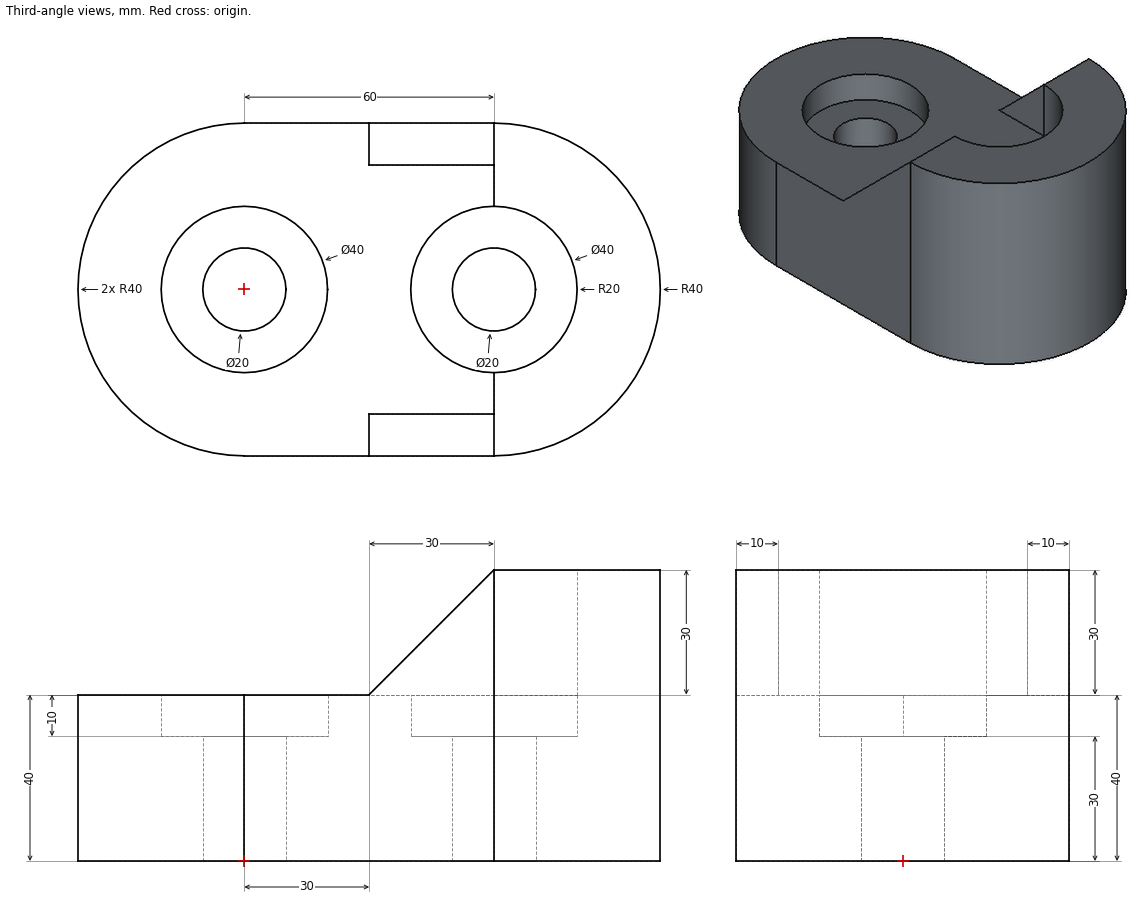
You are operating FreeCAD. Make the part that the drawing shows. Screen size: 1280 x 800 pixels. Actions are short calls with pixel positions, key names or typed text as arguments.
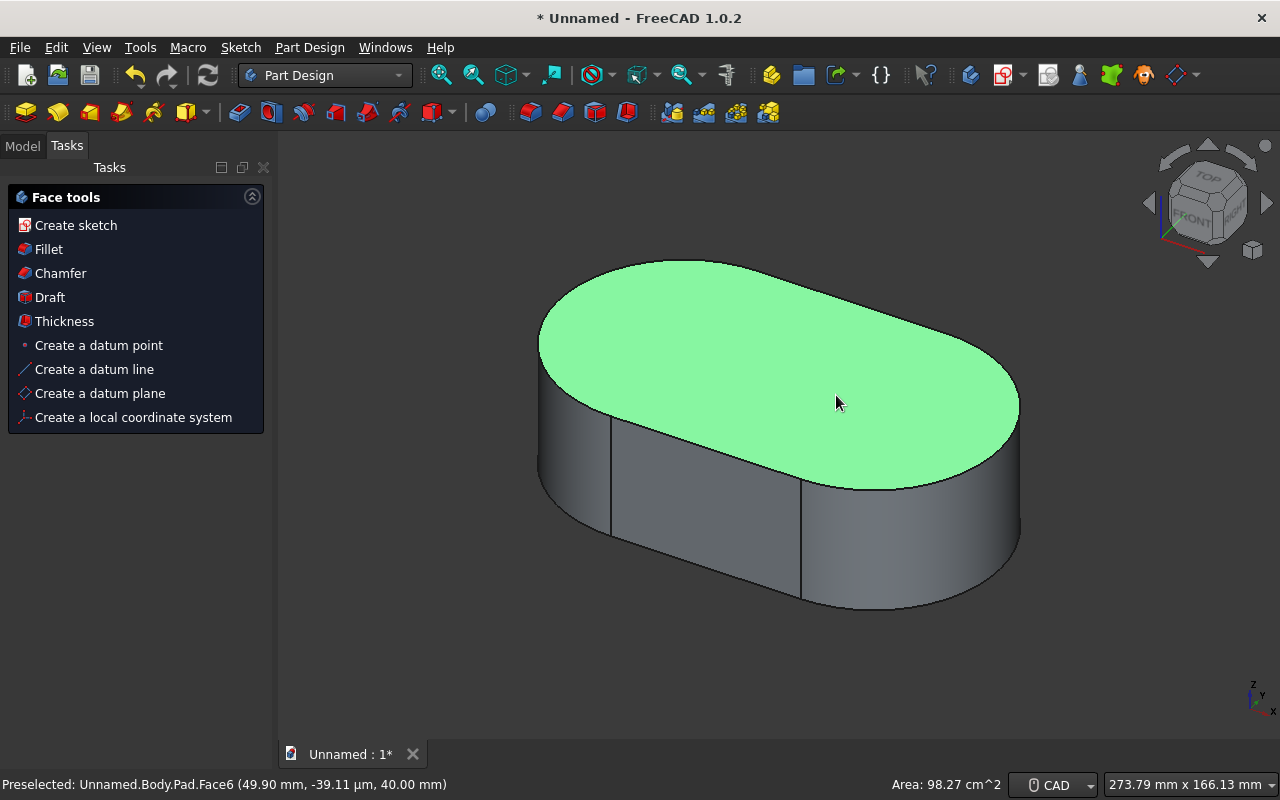
click(1004, 76)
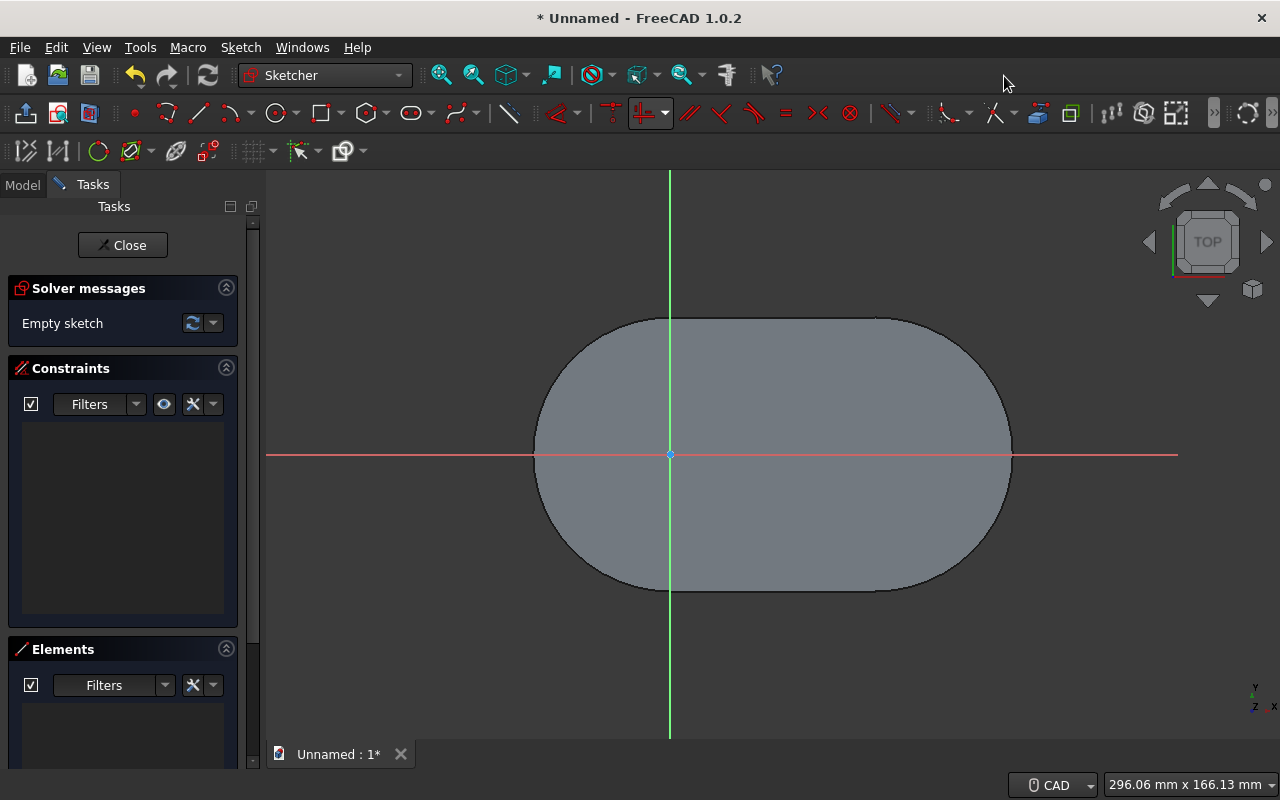
scroll(650, 454, up, 5)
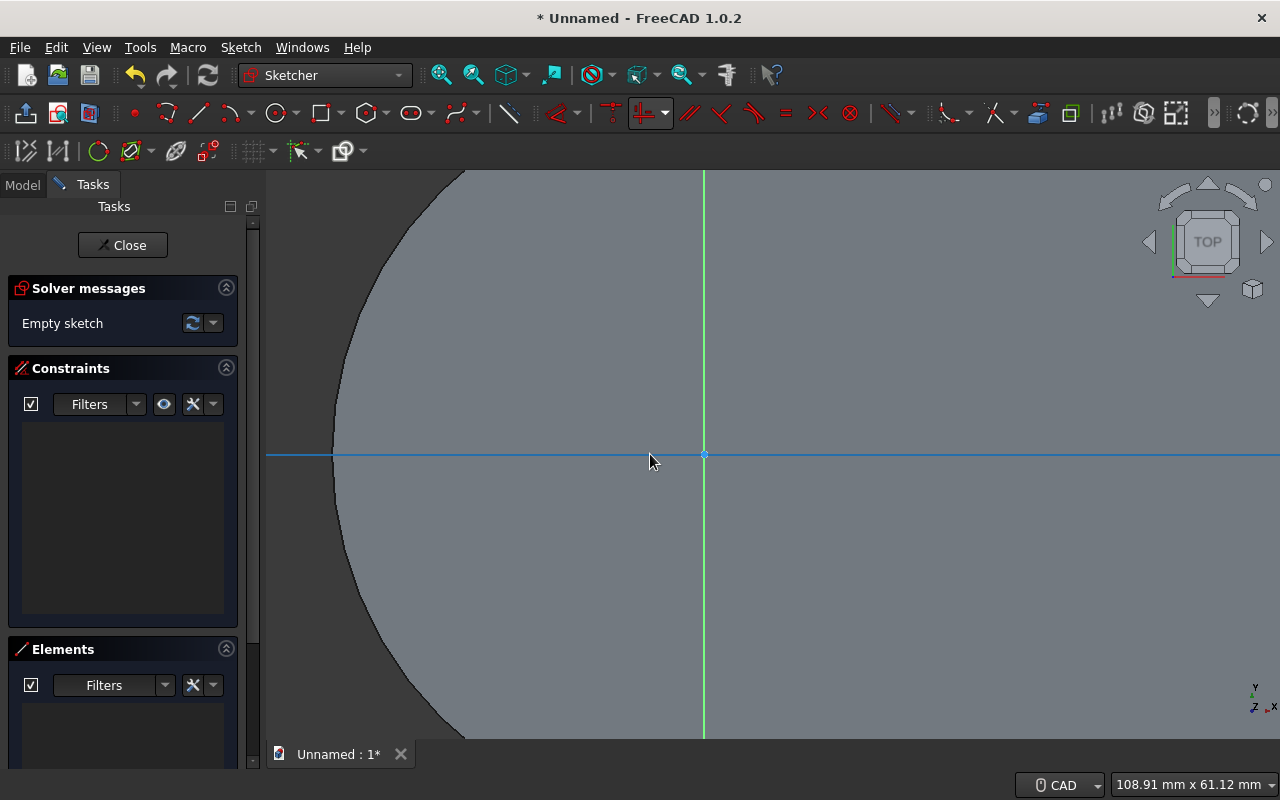
click(276, 114)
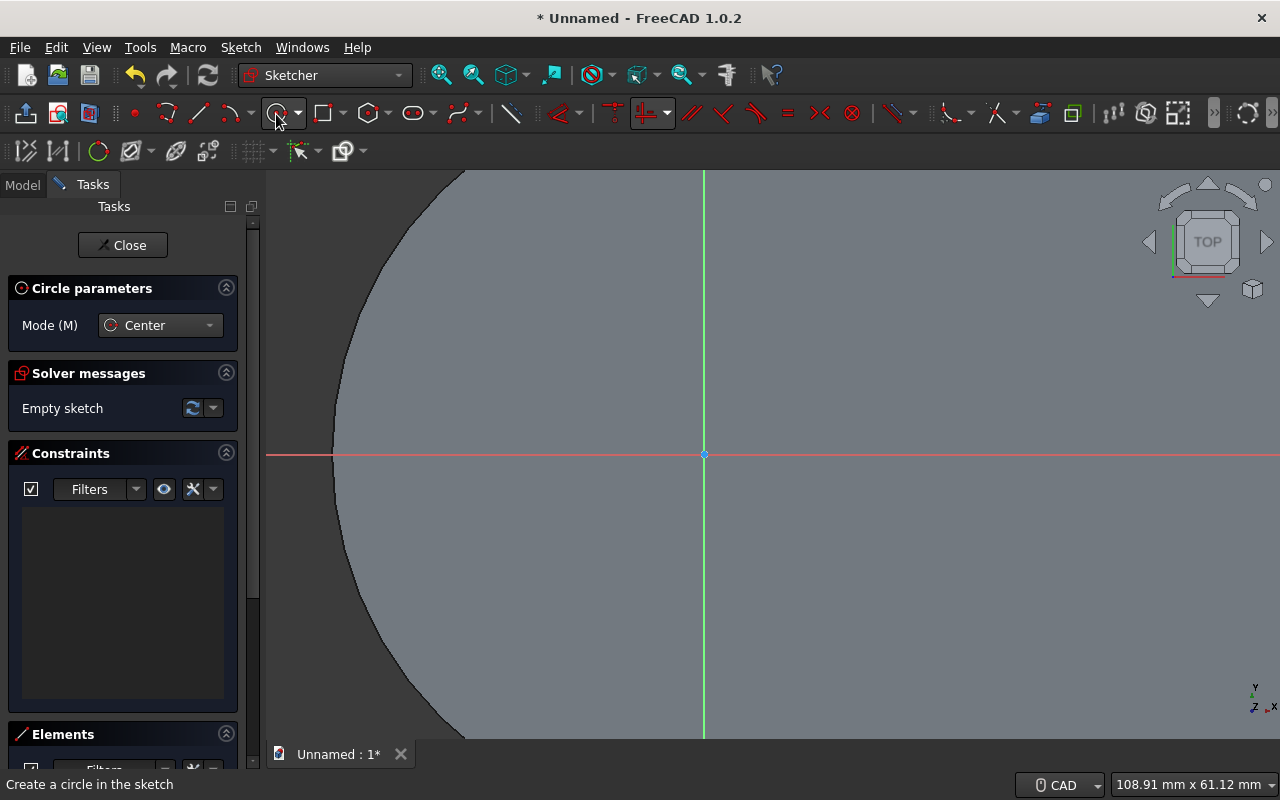
click(704, 454)
move(836, 323)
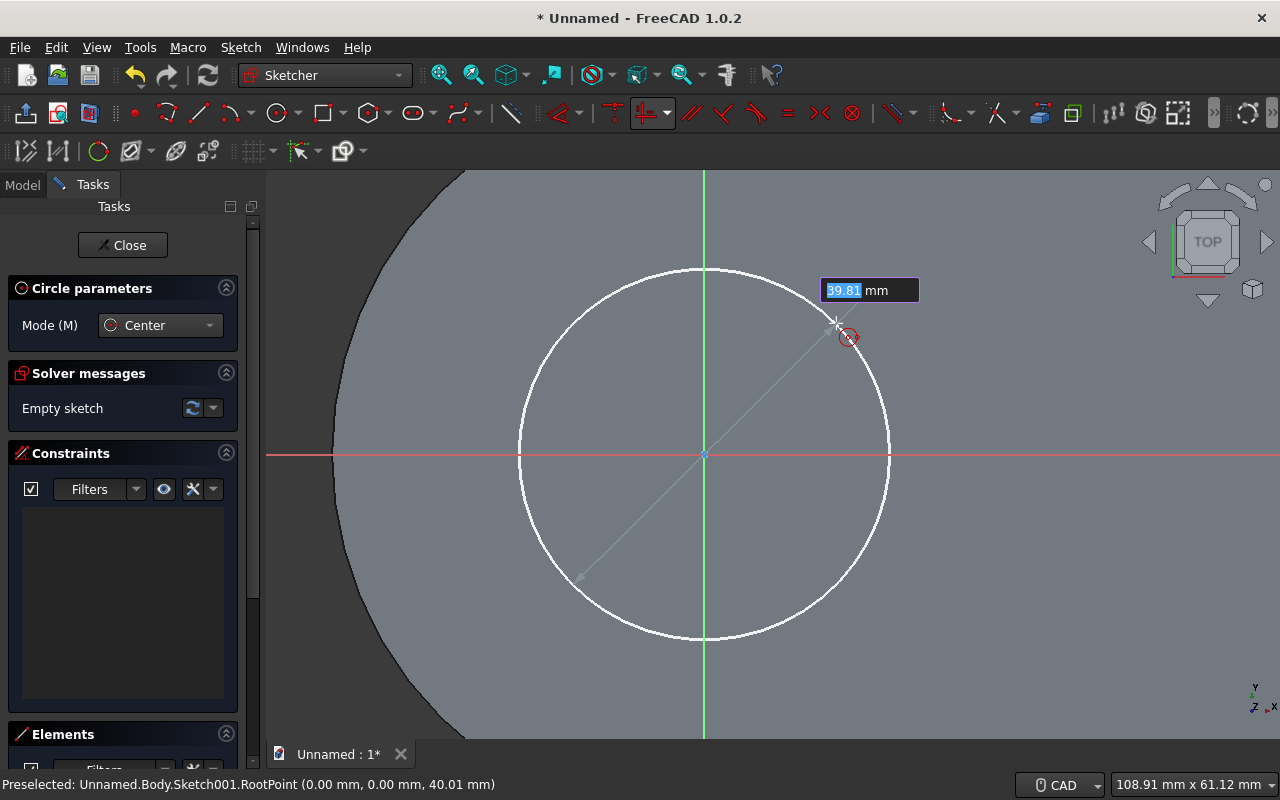
text(40)
key(Return)
key(Escape)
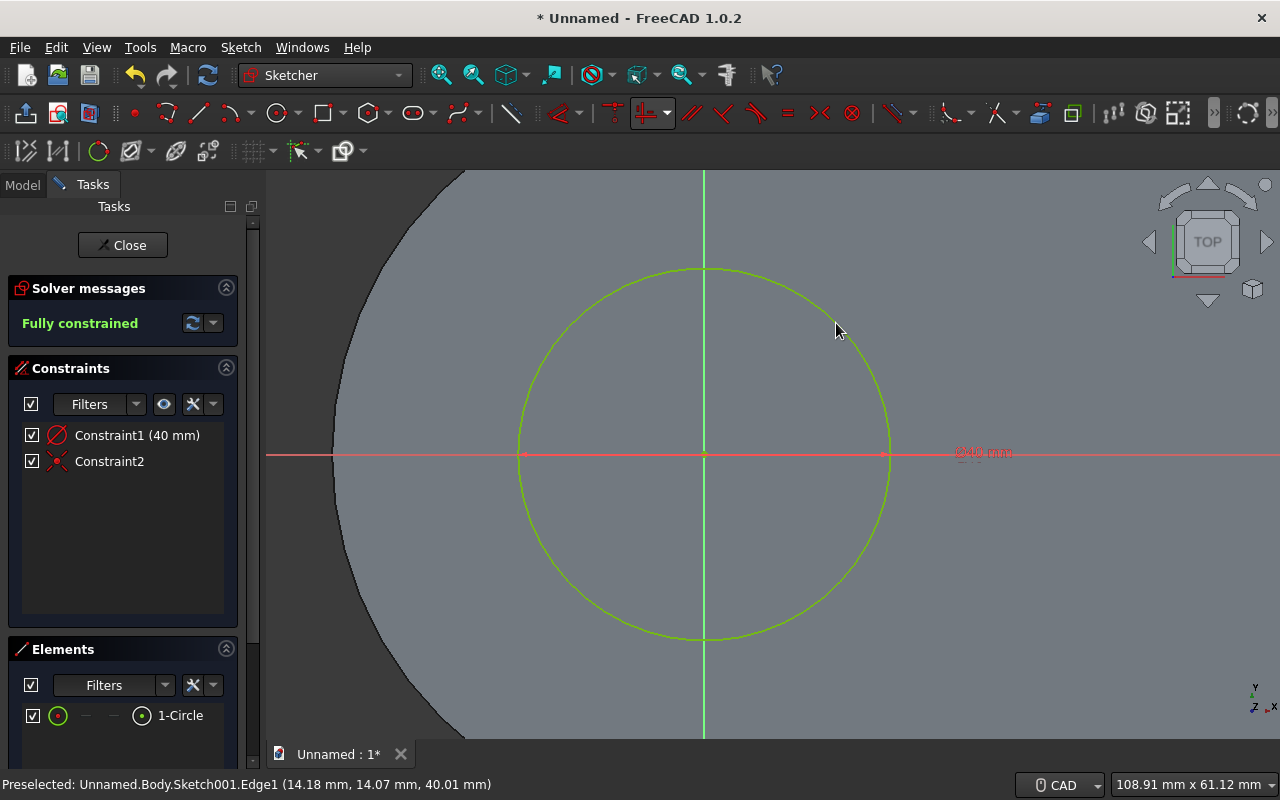
click(123, 245)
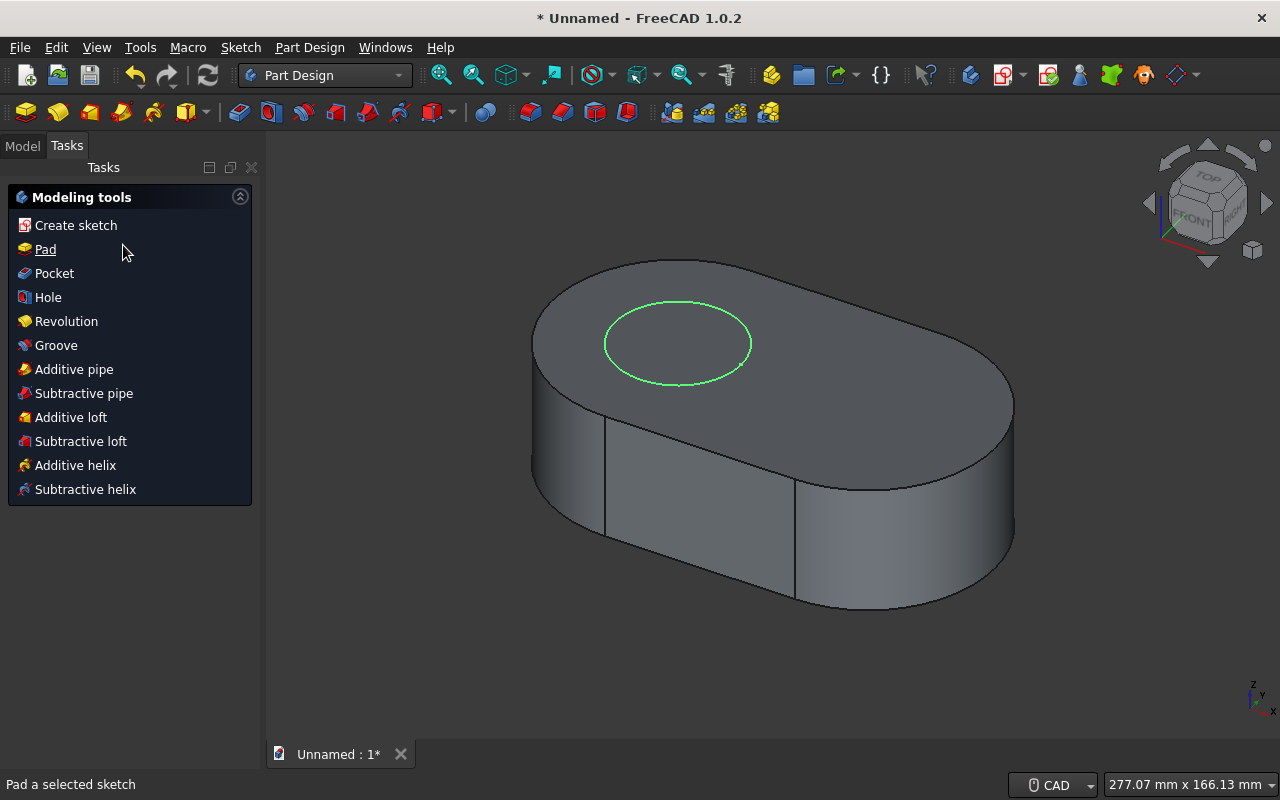
click(240, 112)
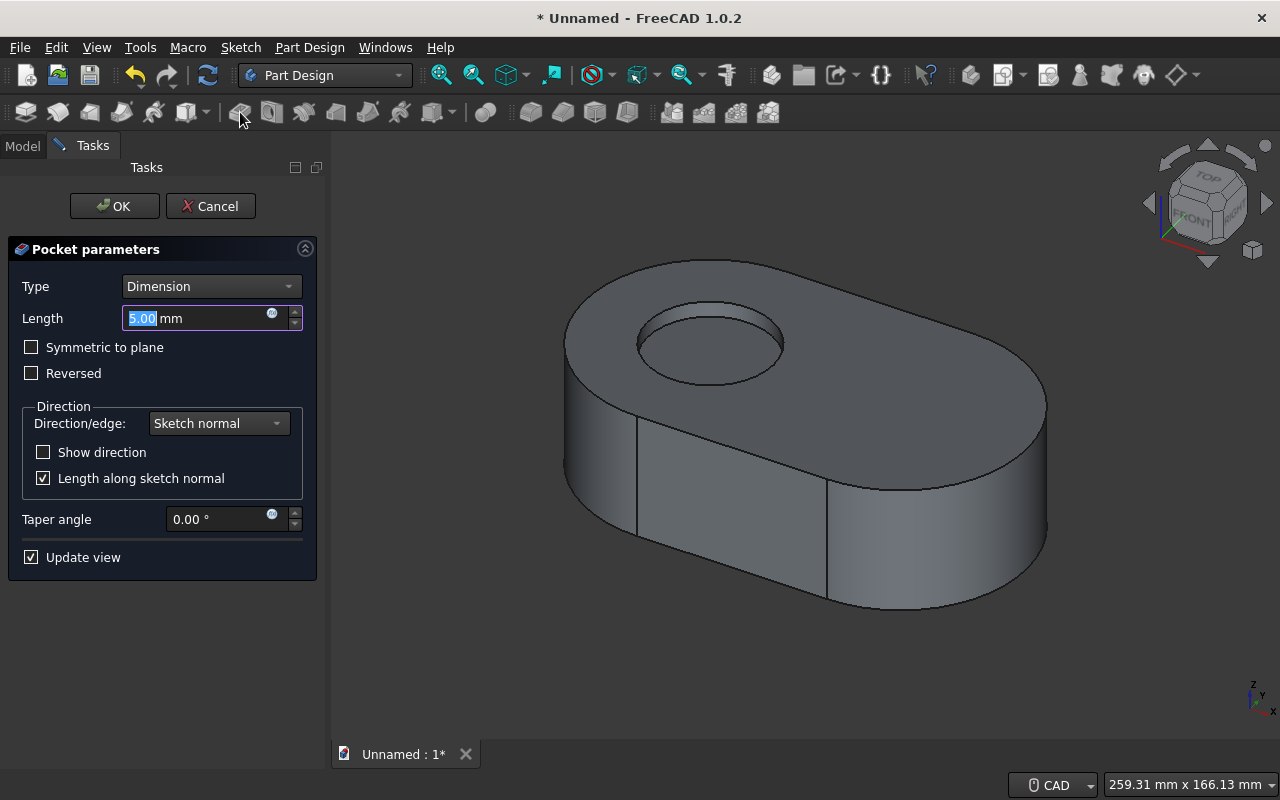
text(10)
key(Tab)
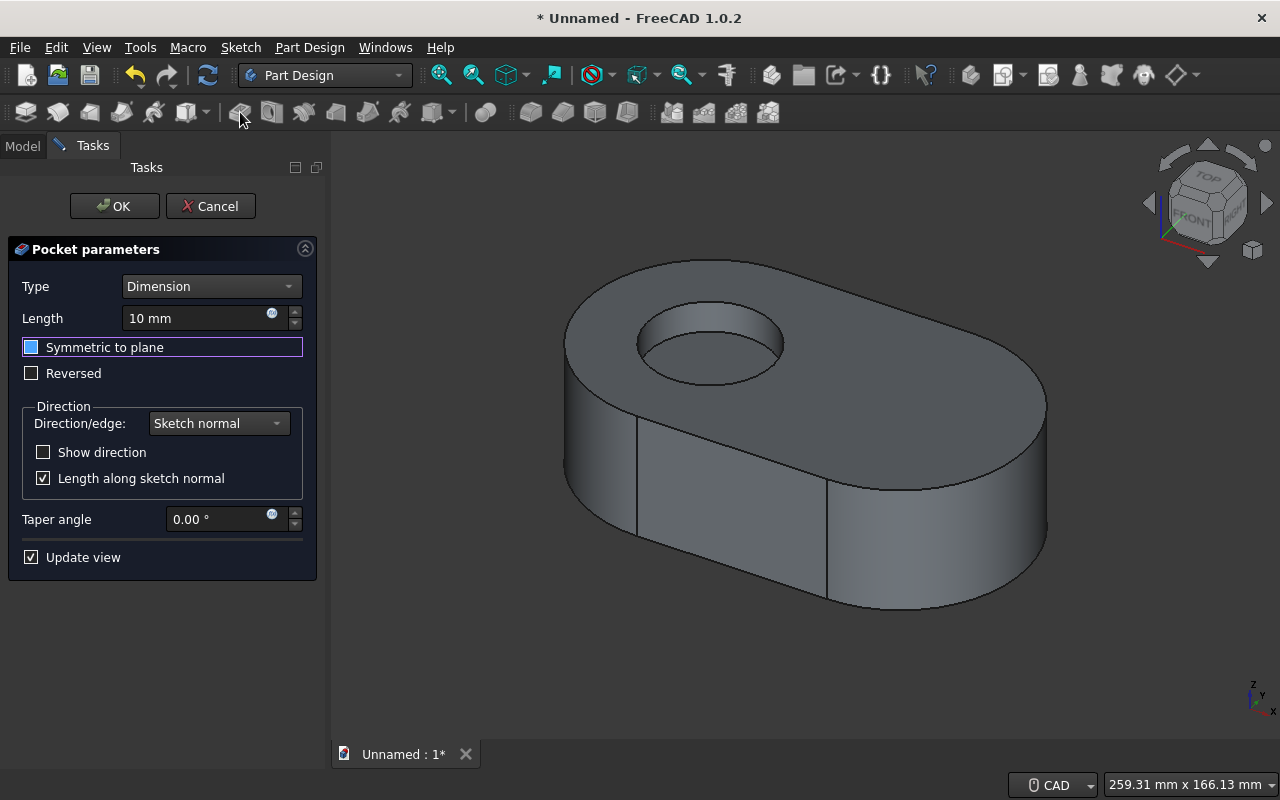
click(115, 206)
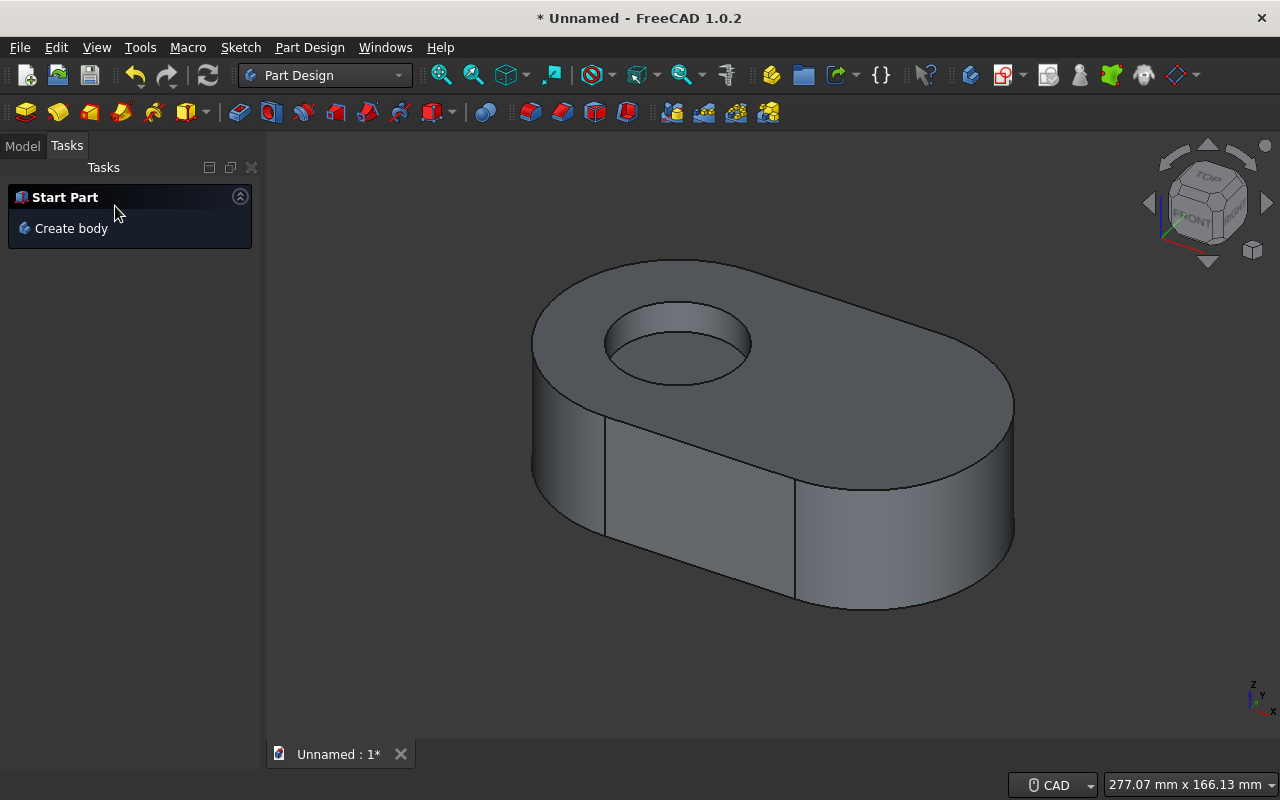
click(678, 373)